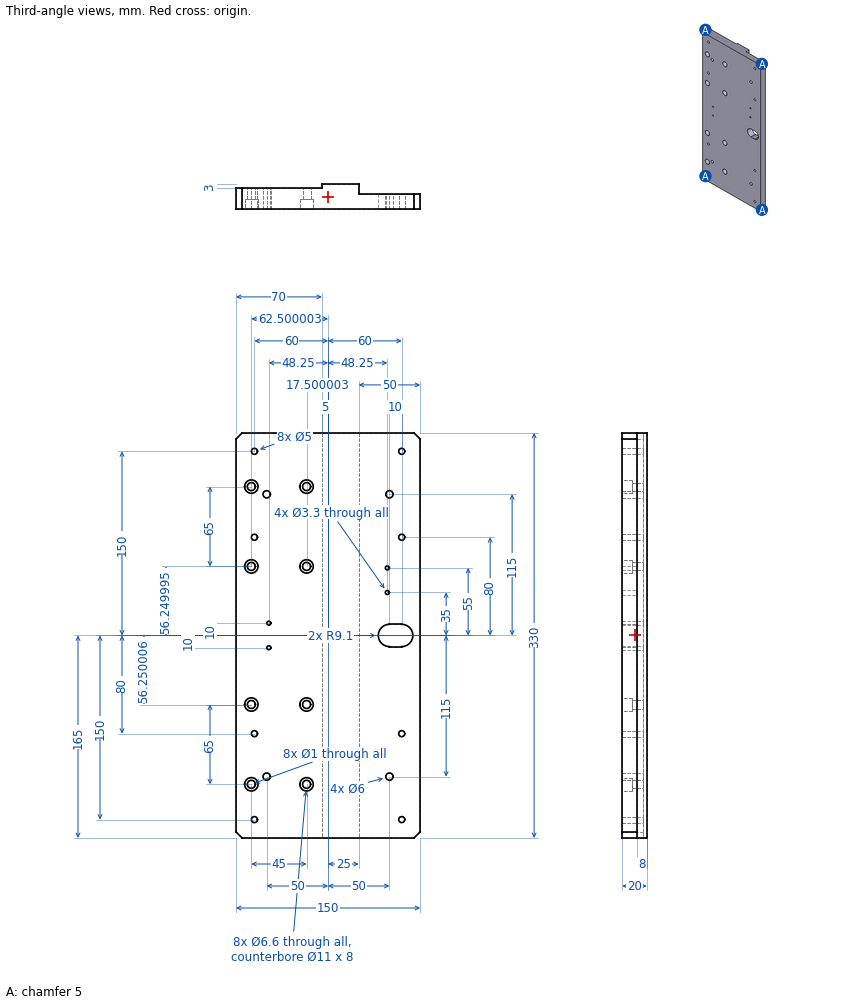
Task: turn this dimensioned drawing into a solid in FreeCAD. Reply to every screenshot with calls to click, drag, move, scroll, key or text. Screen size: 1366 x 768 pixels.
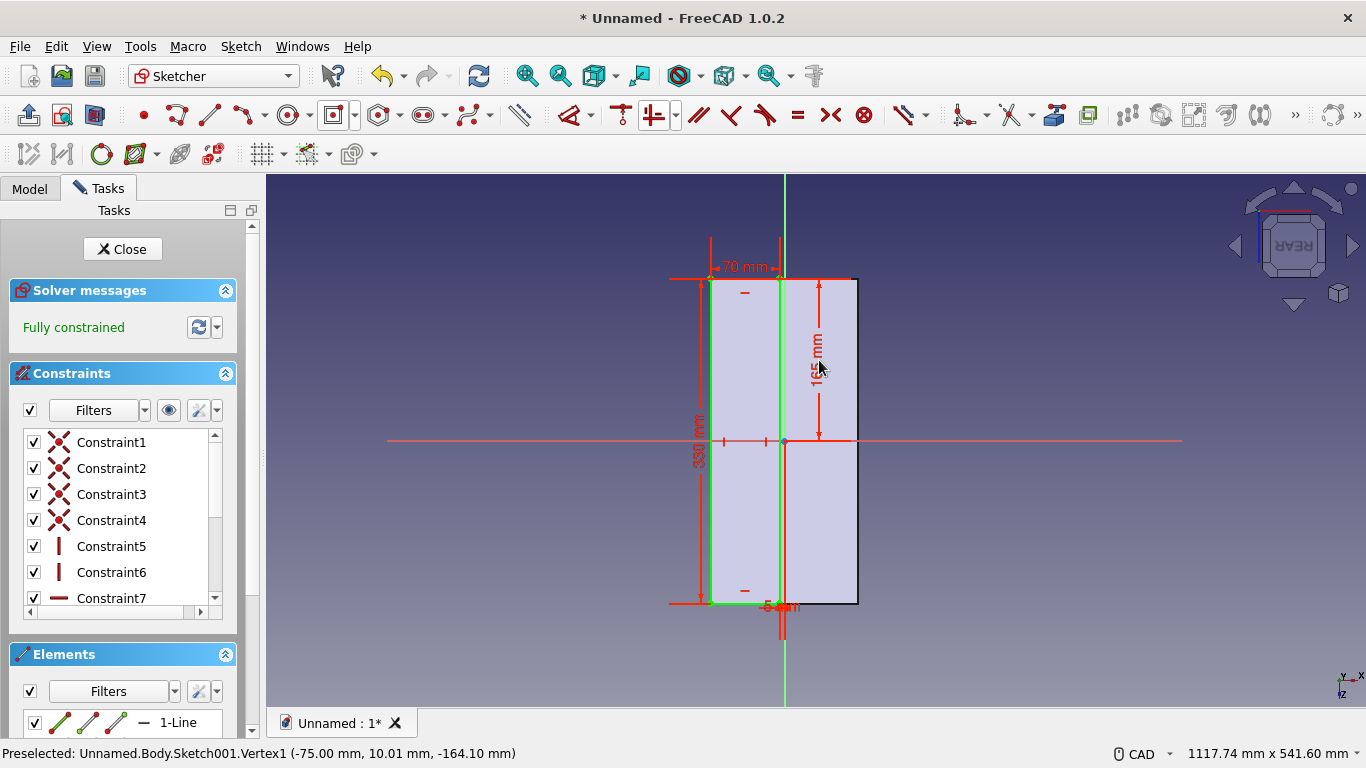
click(123, 249)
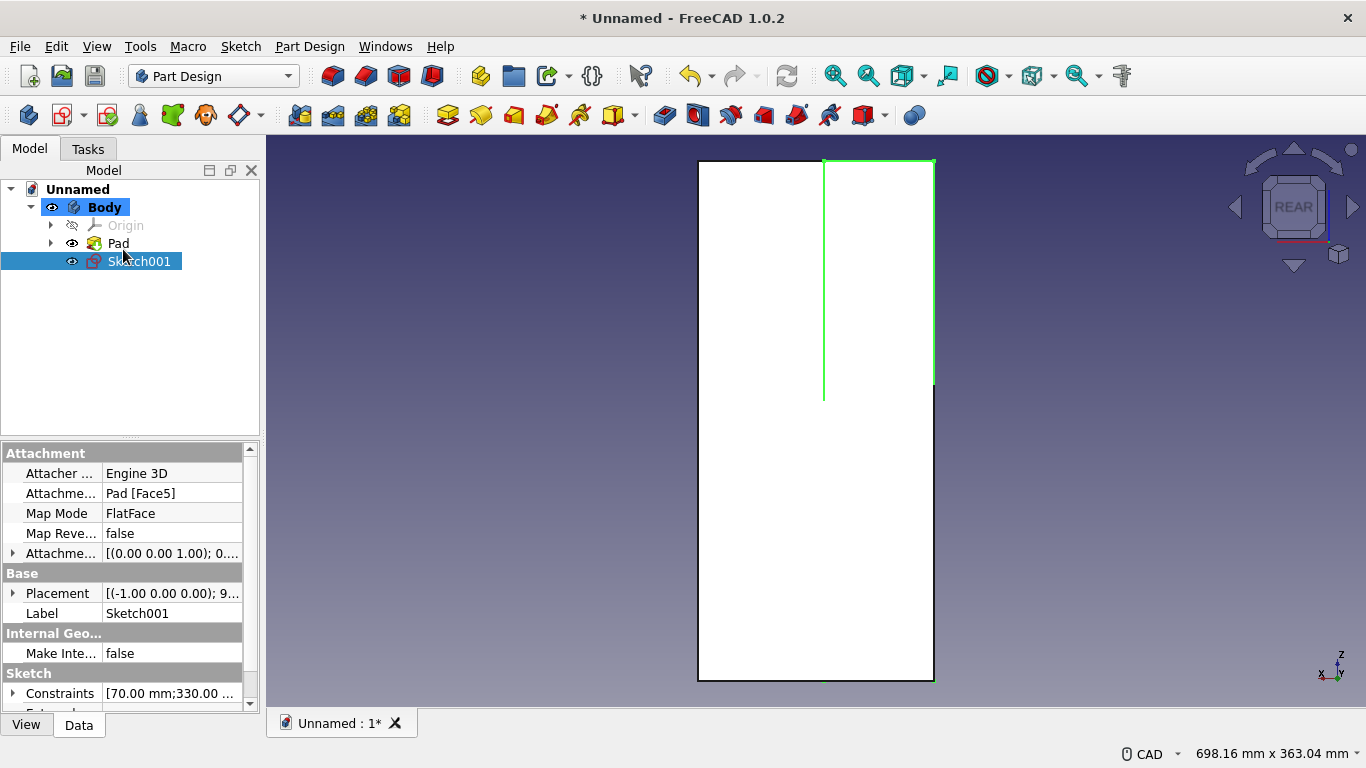
click(665, 116)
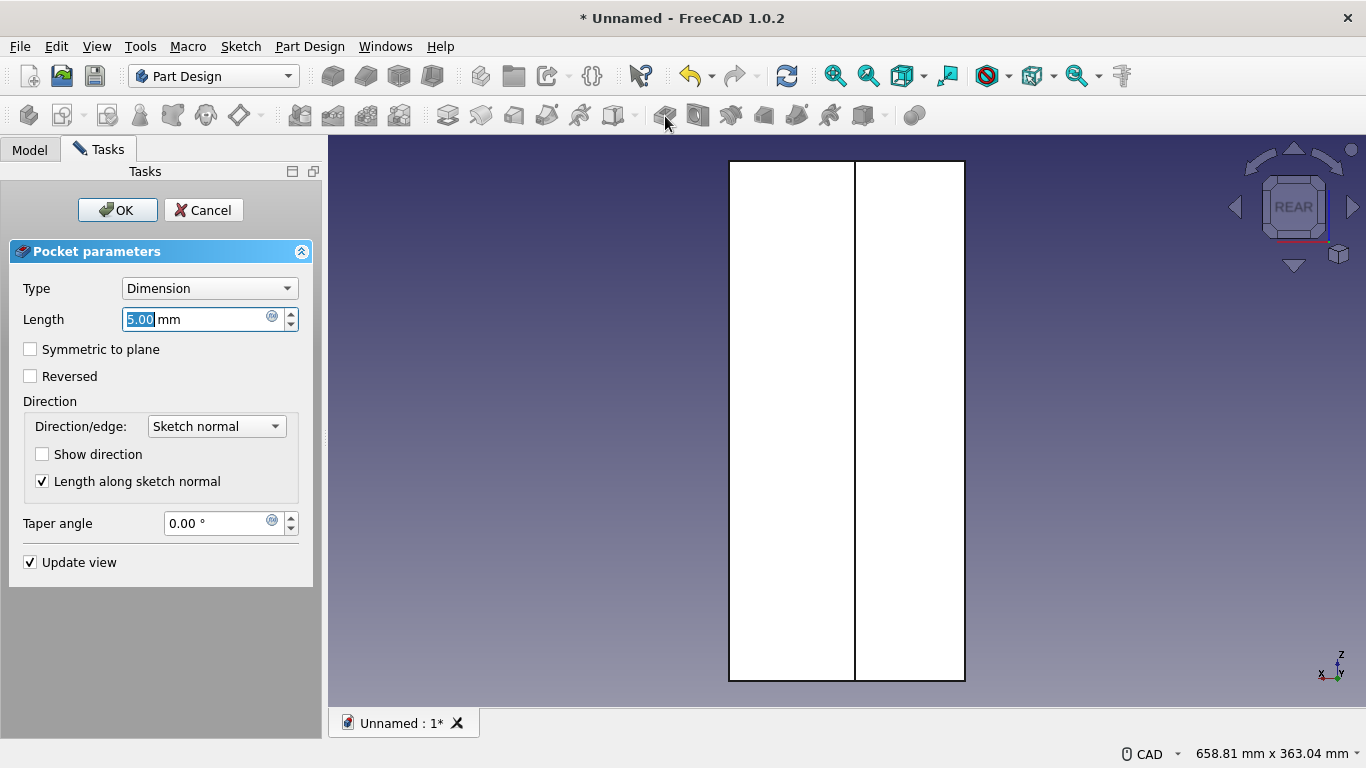
text(3)
key(Tab)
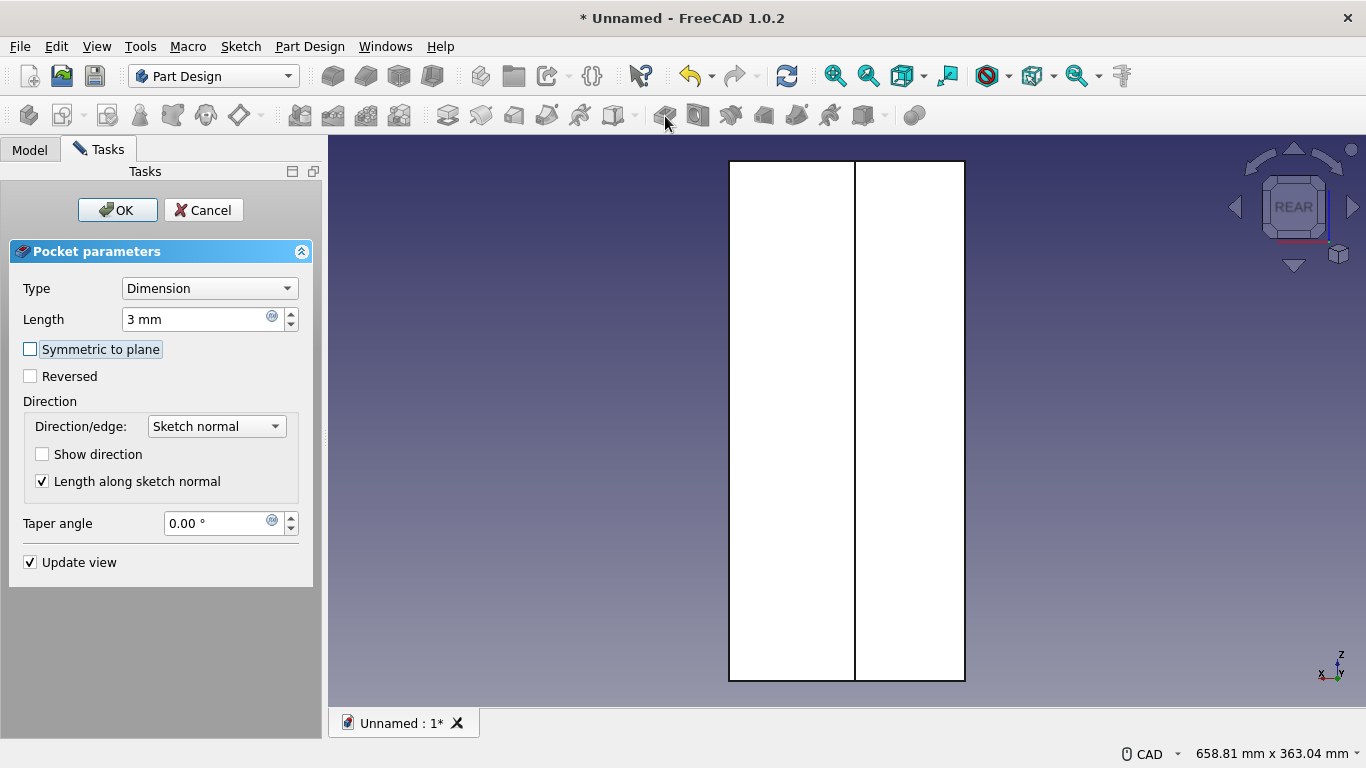
click(118, 210)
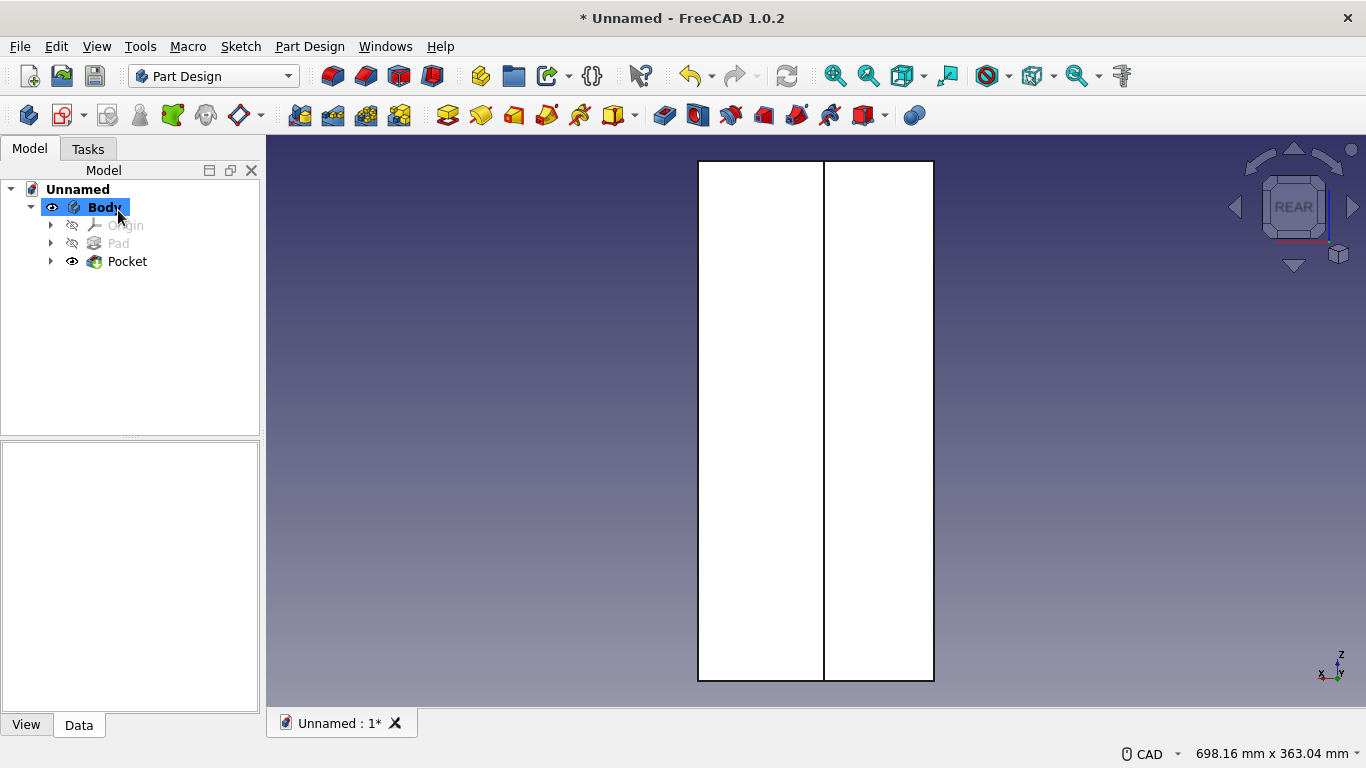
click(761, 271)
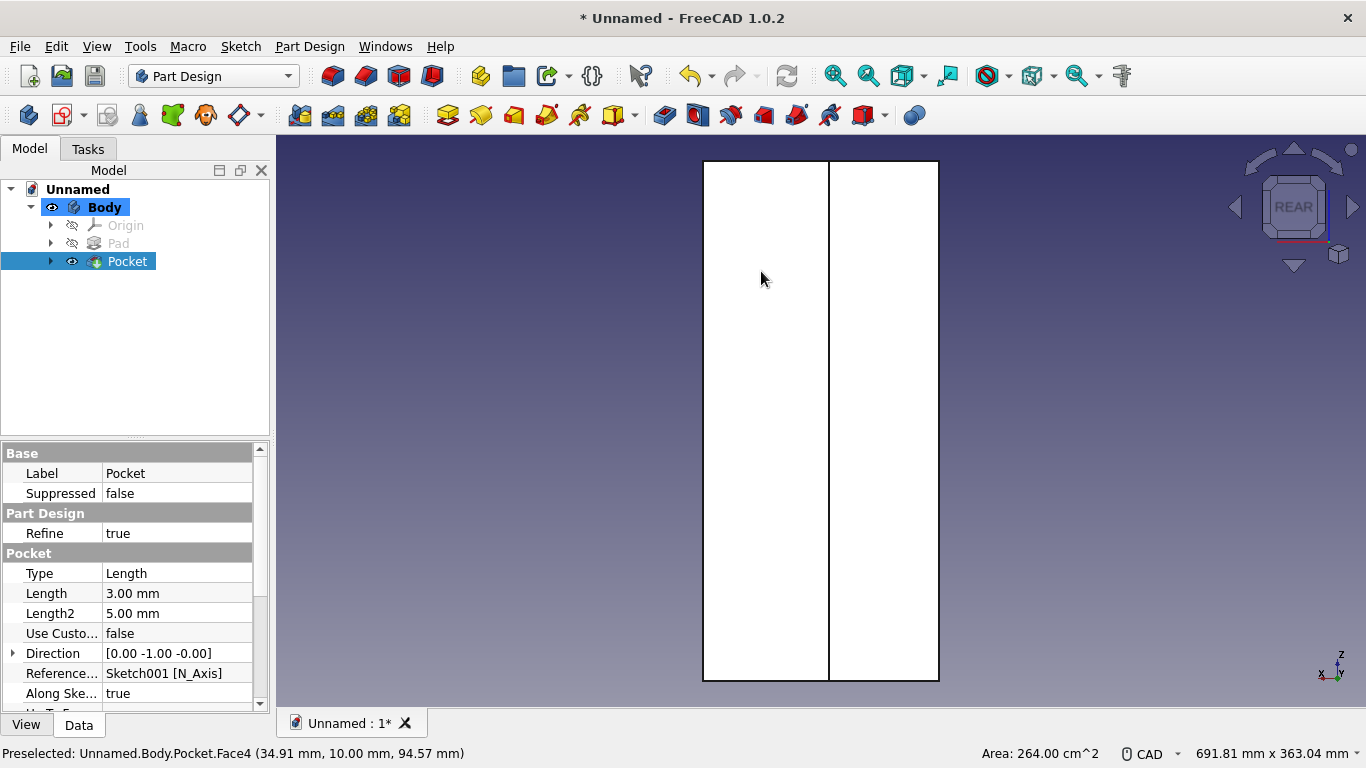
click(62, 116)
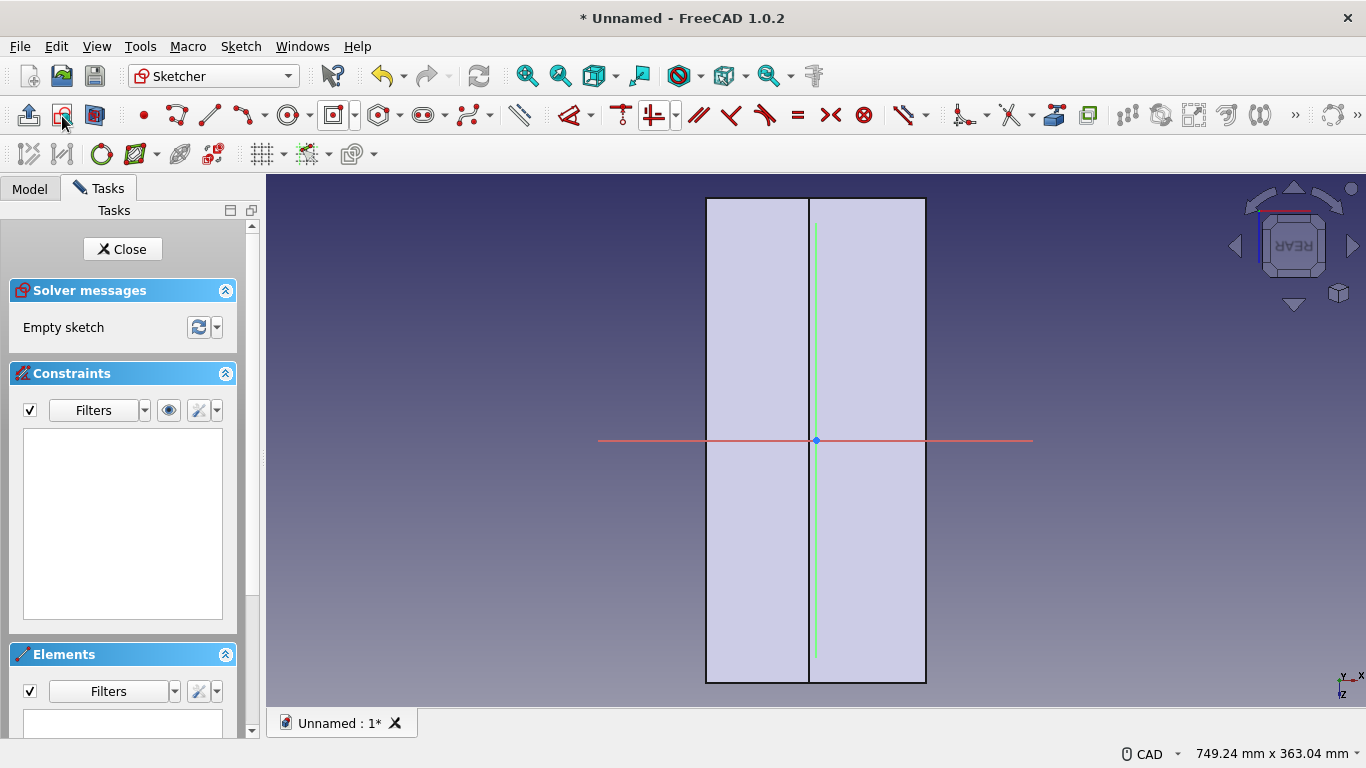
scroll(496, 441, down, 2)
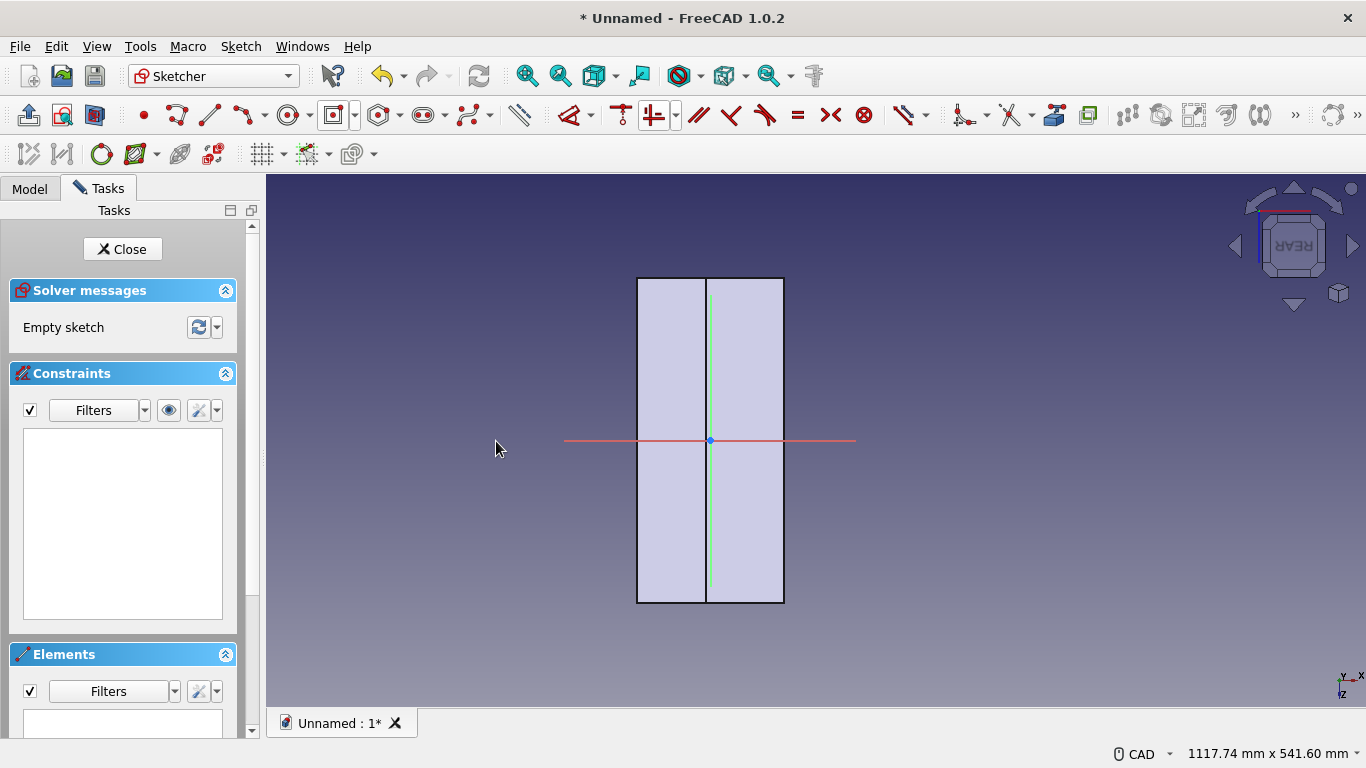
key(g)
key(r)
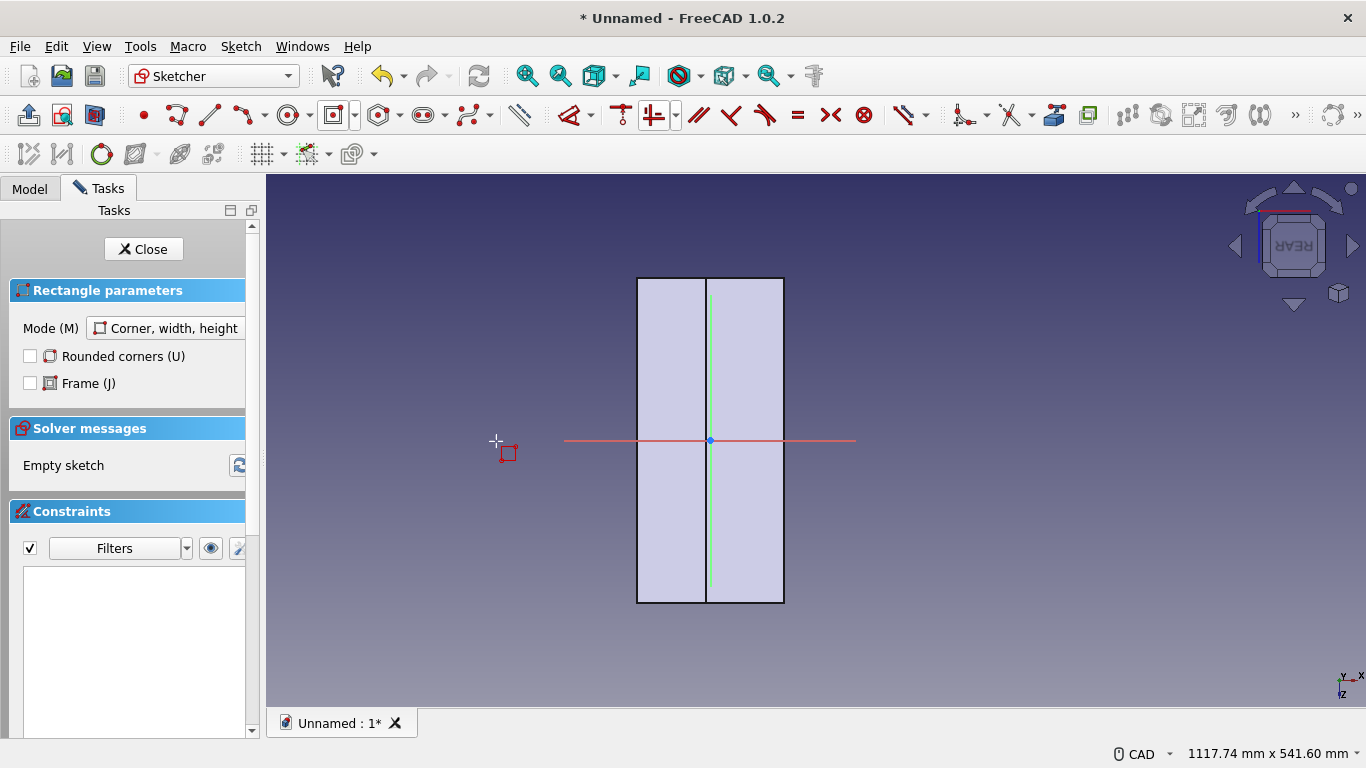
click(735, 278)
move(784, 603)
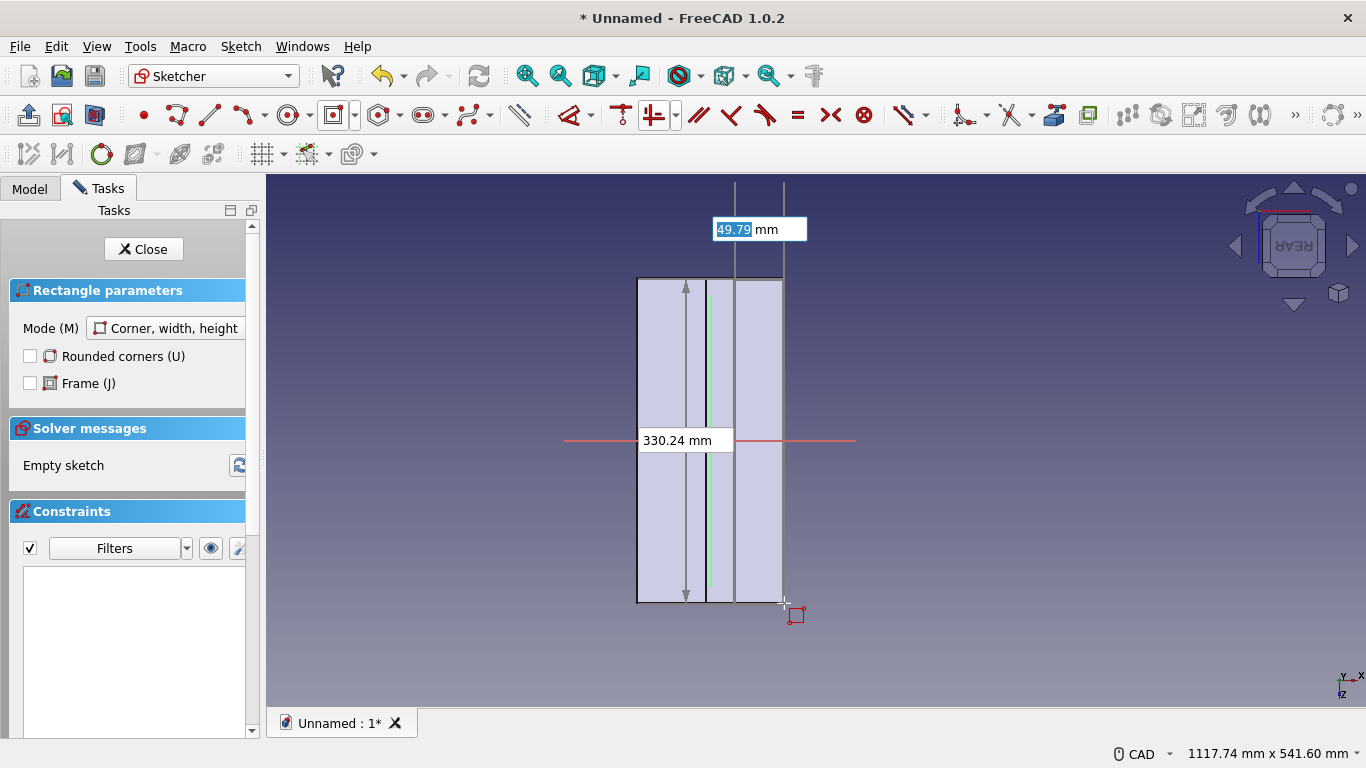
text(50)
key(Tab)
text(330)
key(Return)
key(Escape)